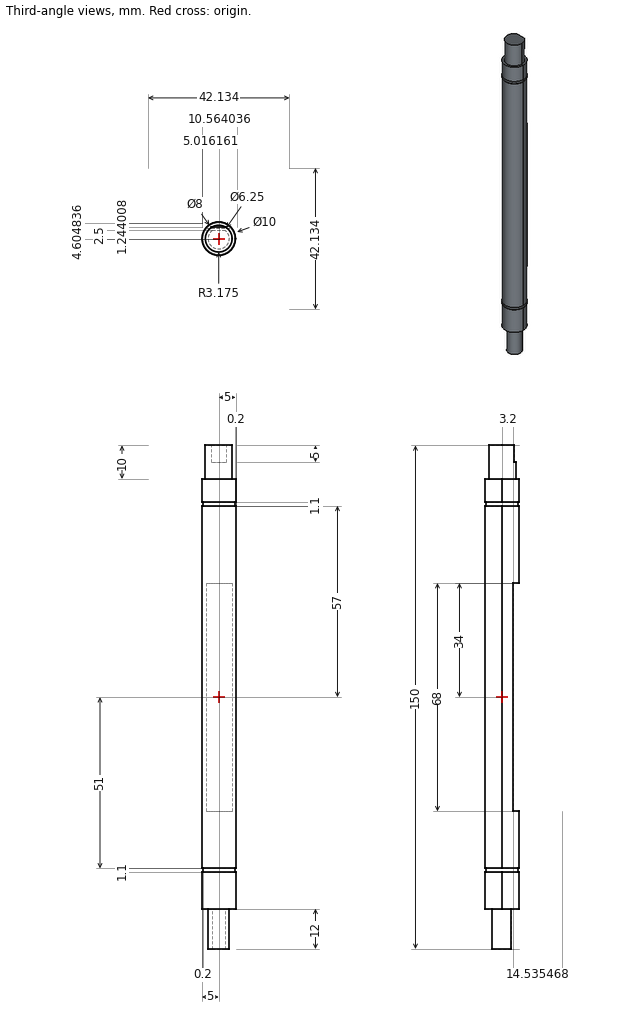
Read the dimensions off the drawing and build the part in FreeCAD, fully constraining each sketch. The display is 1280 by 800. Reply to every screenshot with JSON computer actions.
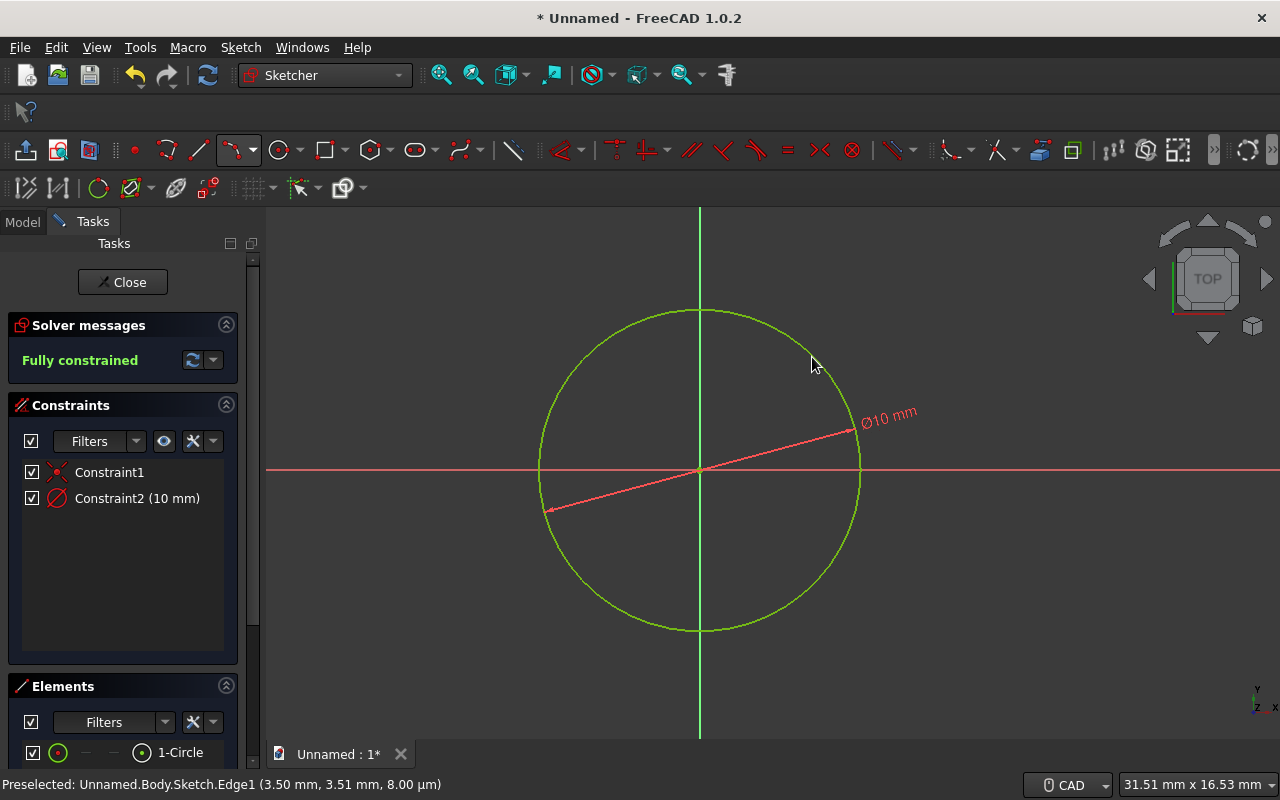
{"action": "left_click", "coordinate": [123, 282]}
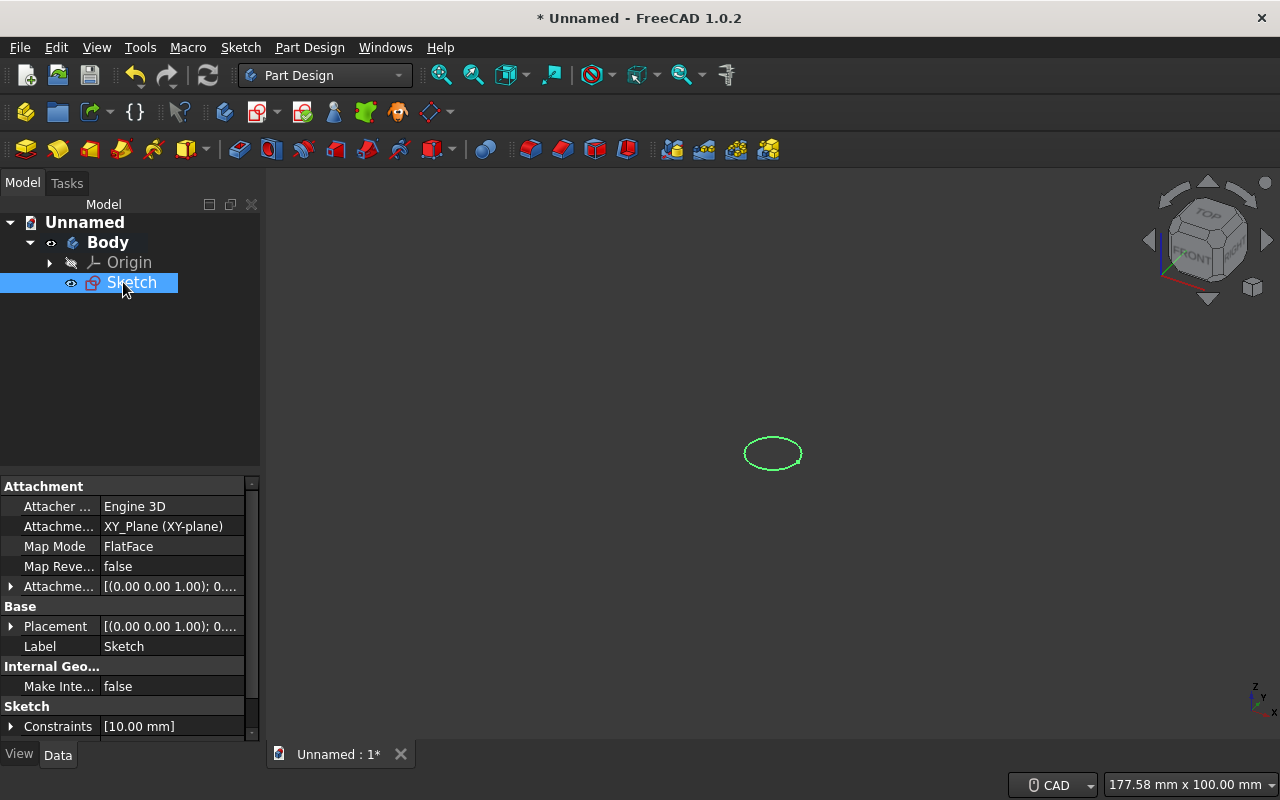
{"action": "left_click", "coordinate": [26, 150]}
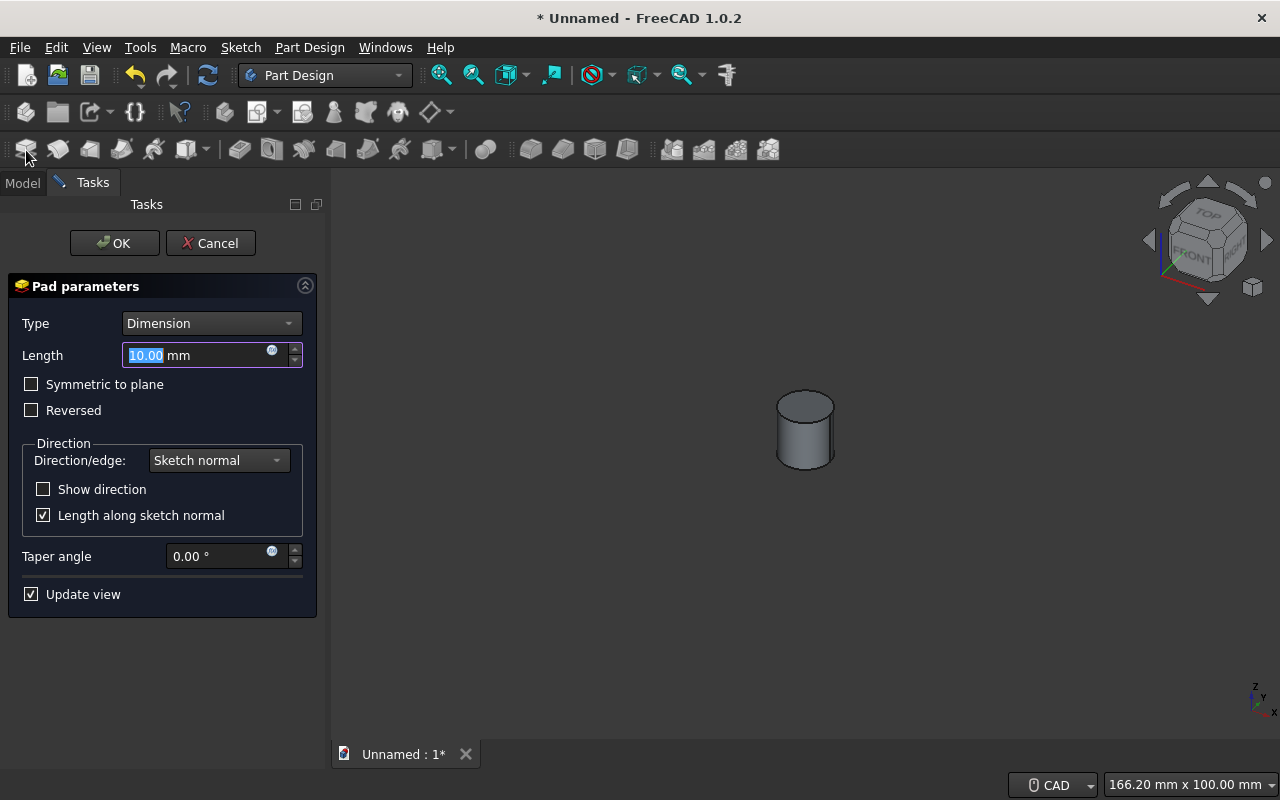
{"action": "type", "text": "150"}
{"action": "key", "text": "Tab"}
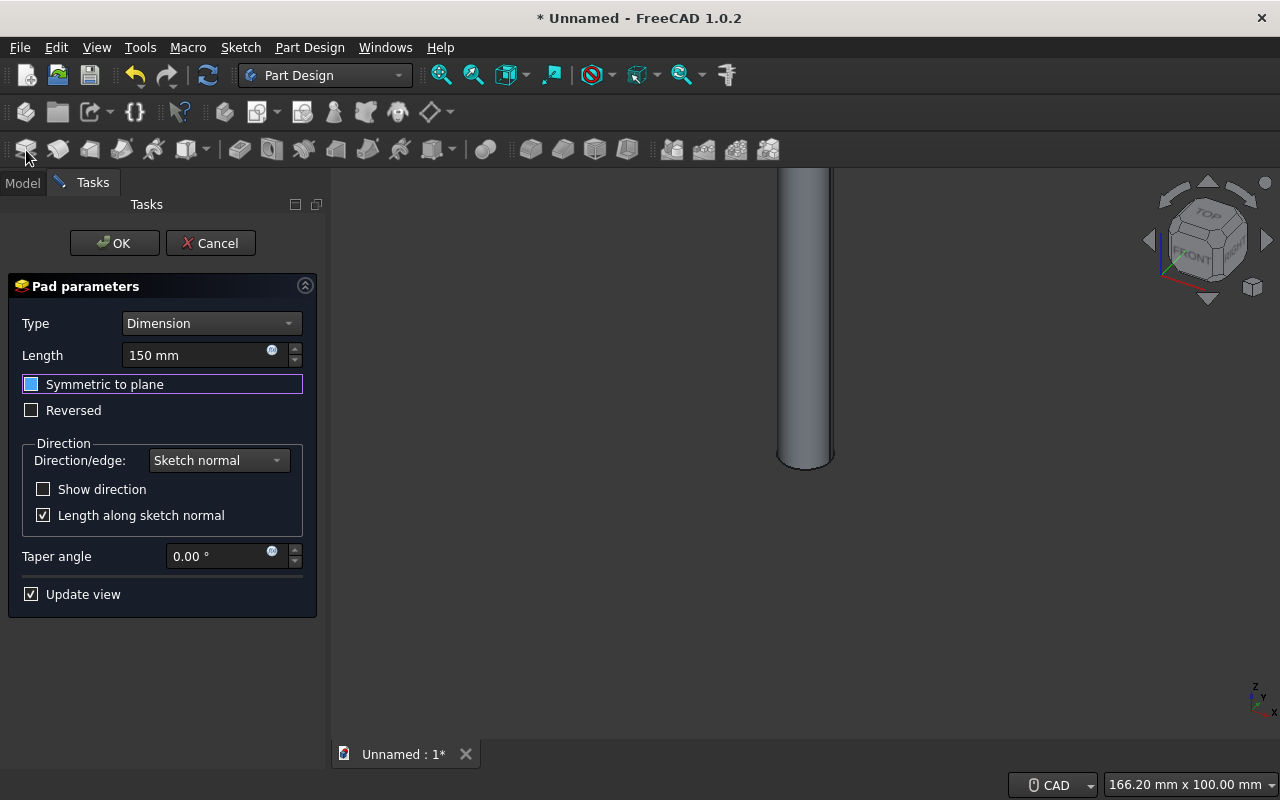
{"action": "left_click", "coordinate": [30, 384]}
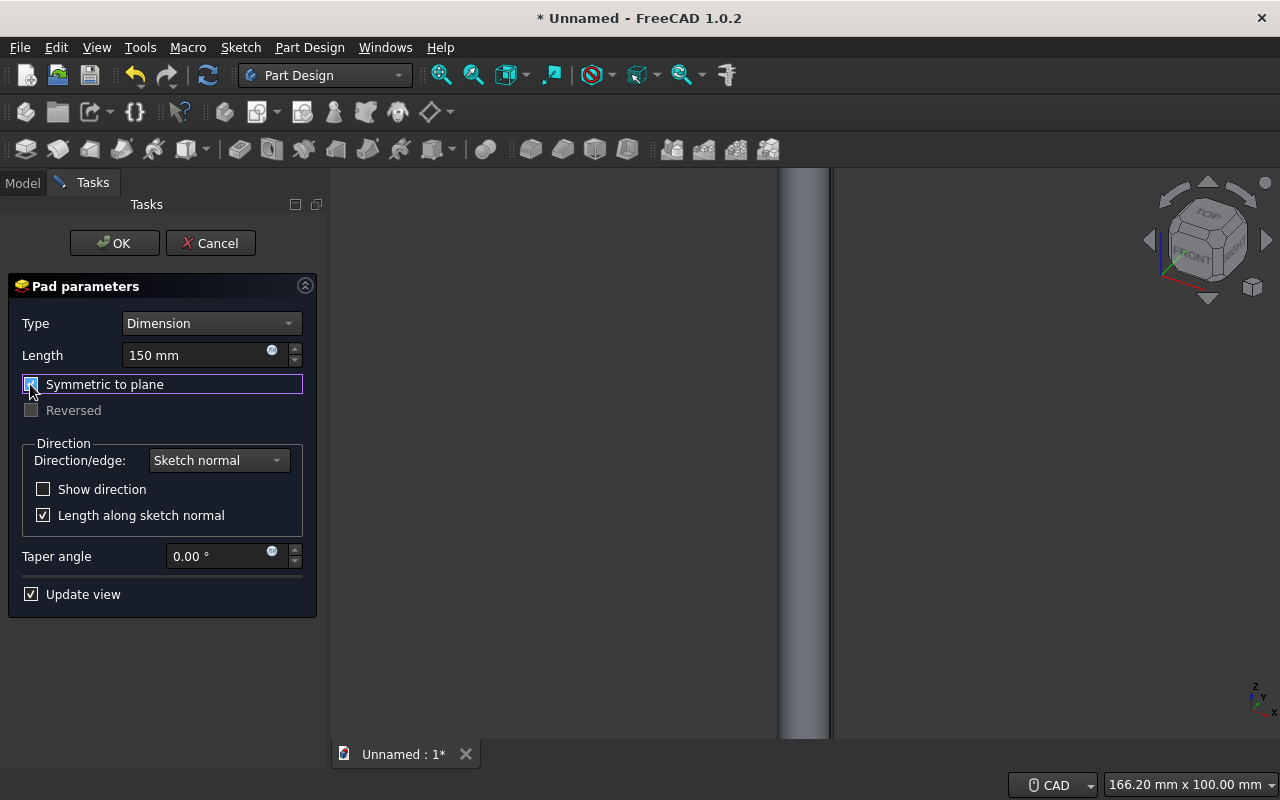
{"action": "left_click", "coordinate": [115, 243]}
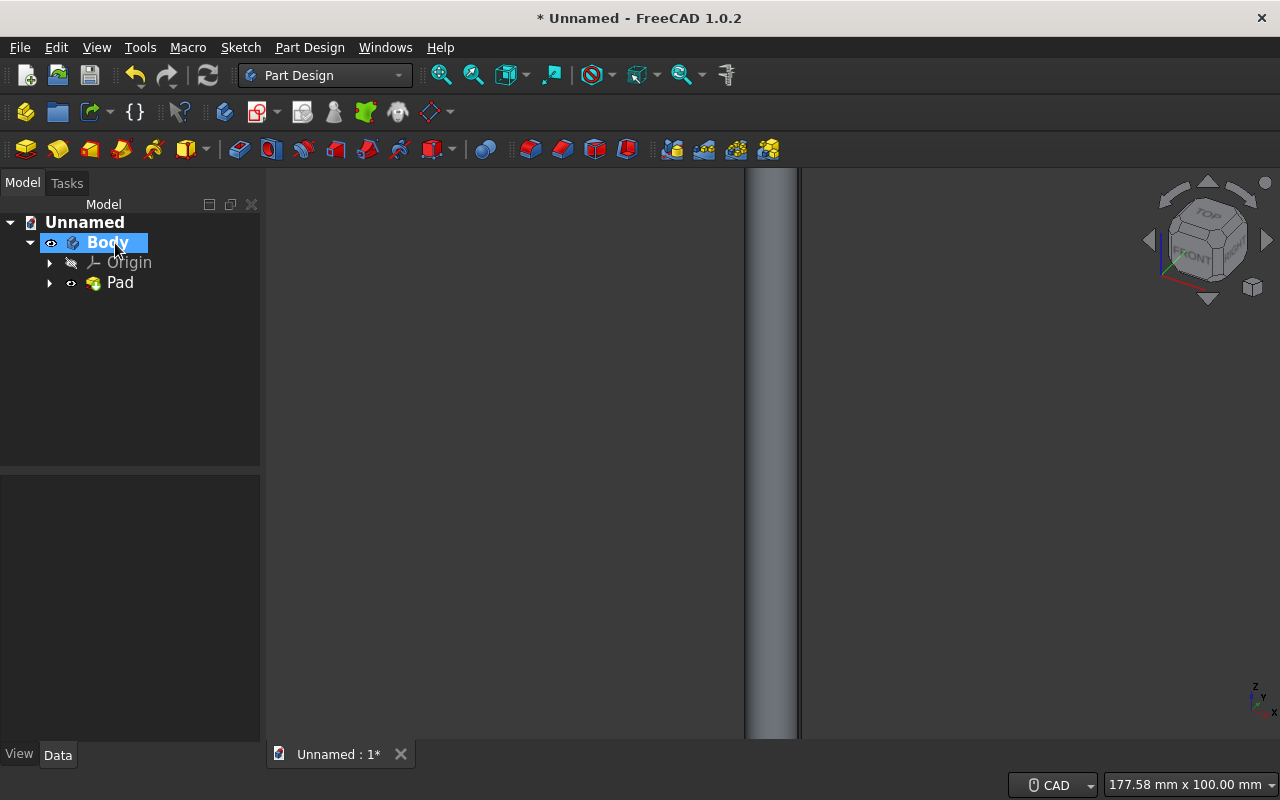
{"action": "left_click", "coordinate": [442, 76]}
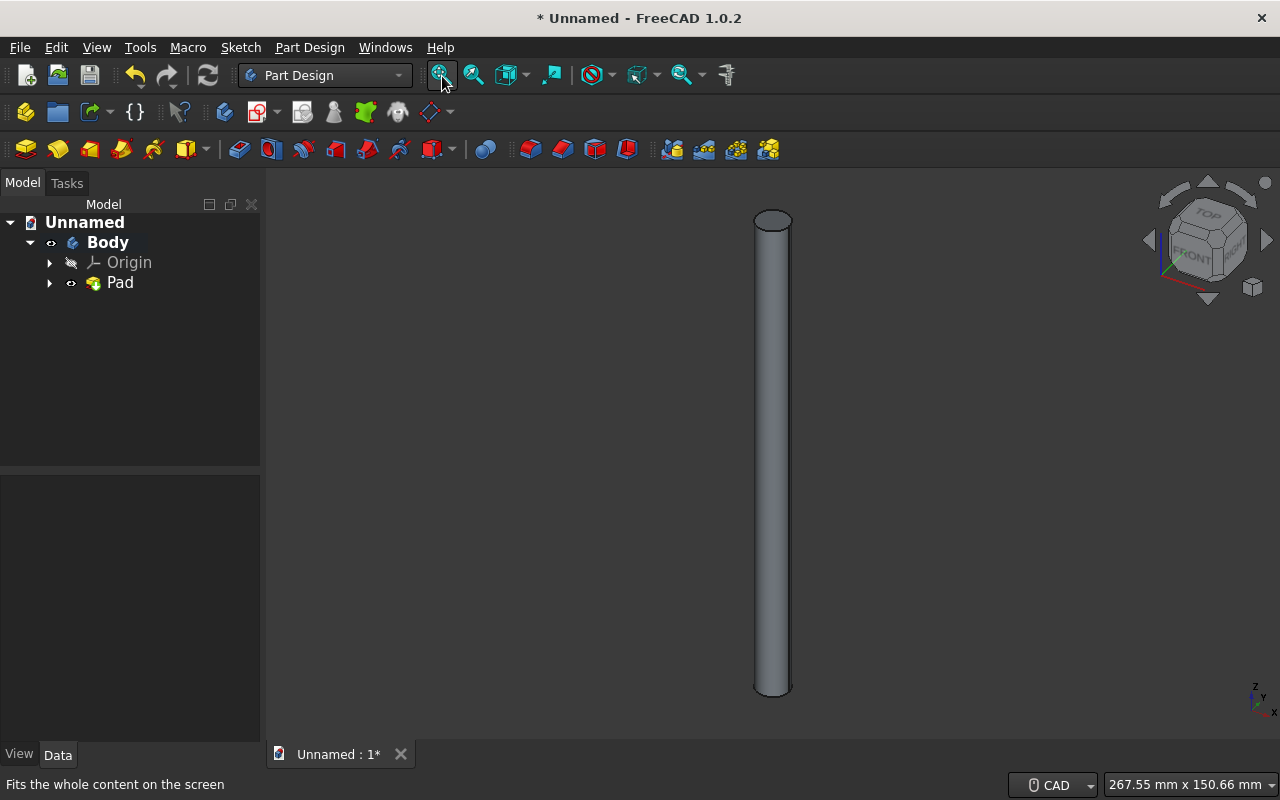
{"action": "left_click", "coordinate": [258, 112]}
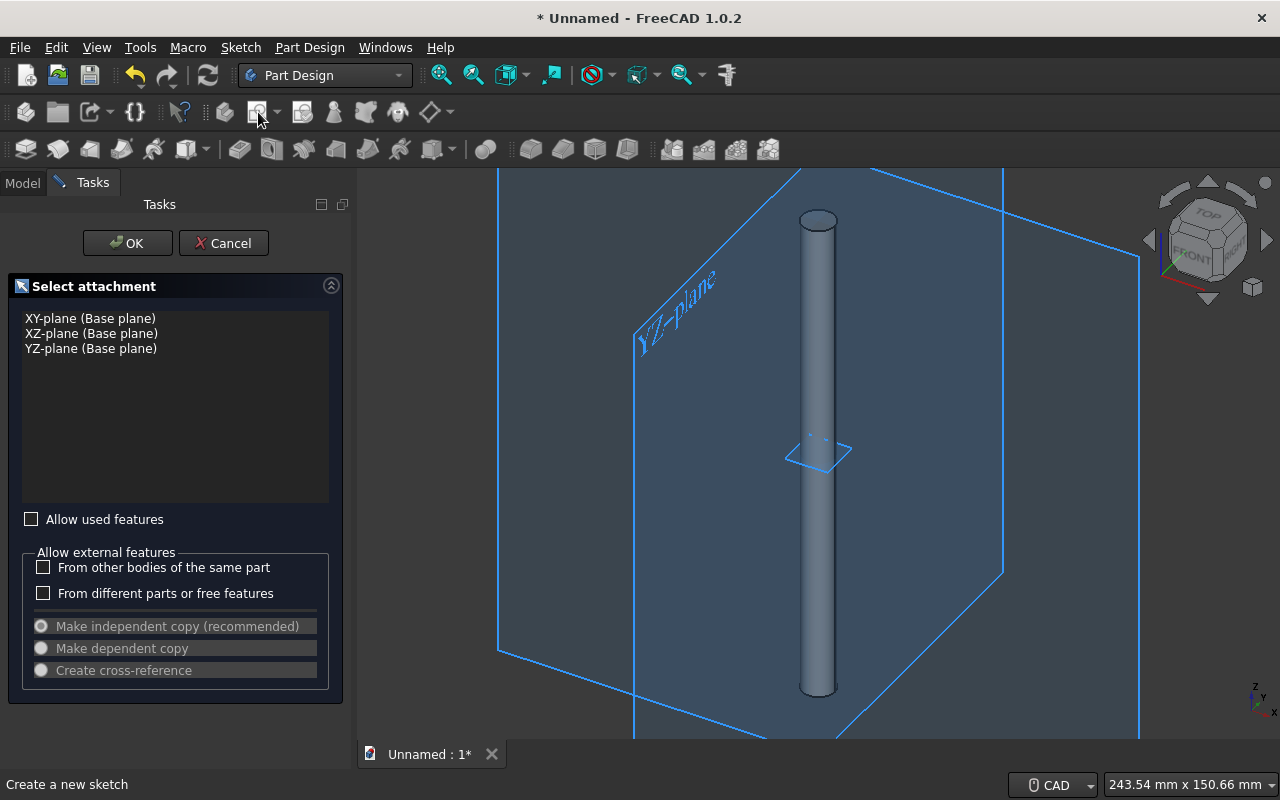
{"action": "left_click", "coordinate": [82, 348]}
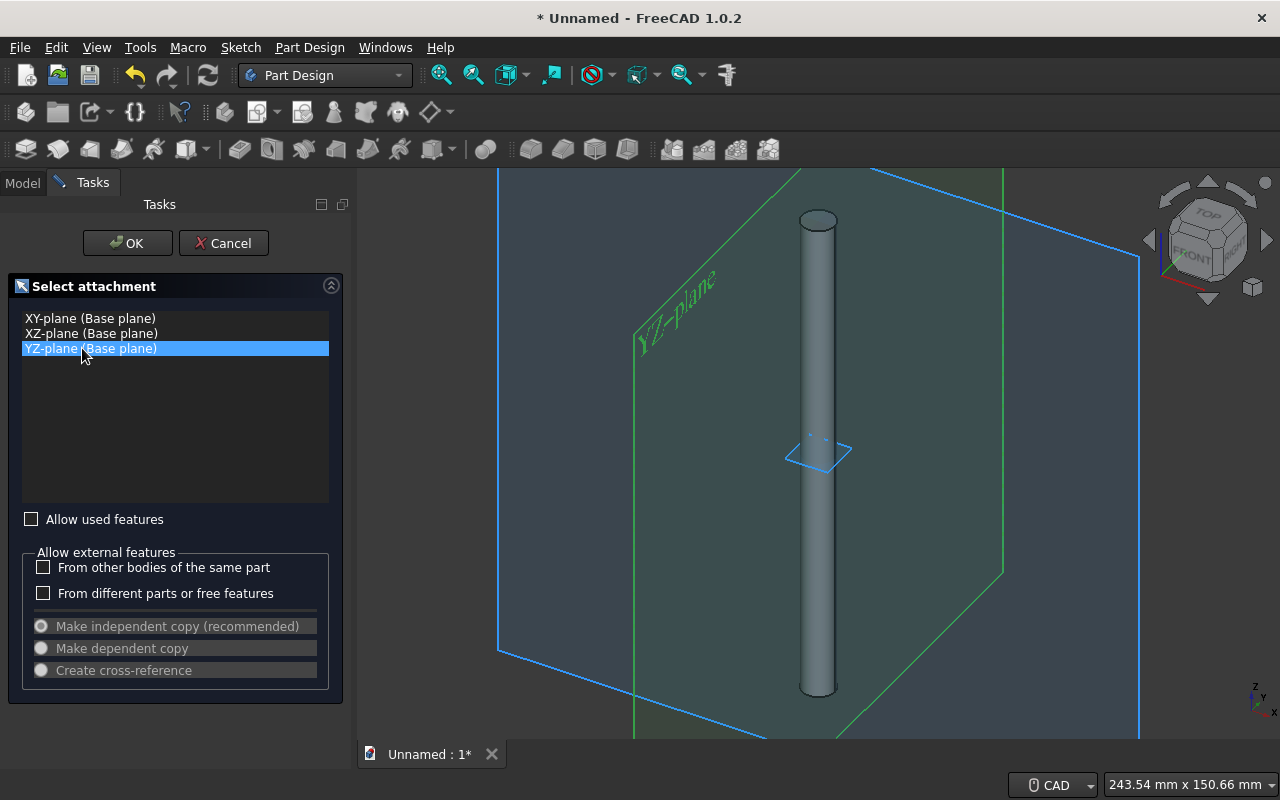
{"action": "left_click", "coordinate": [128, 243]}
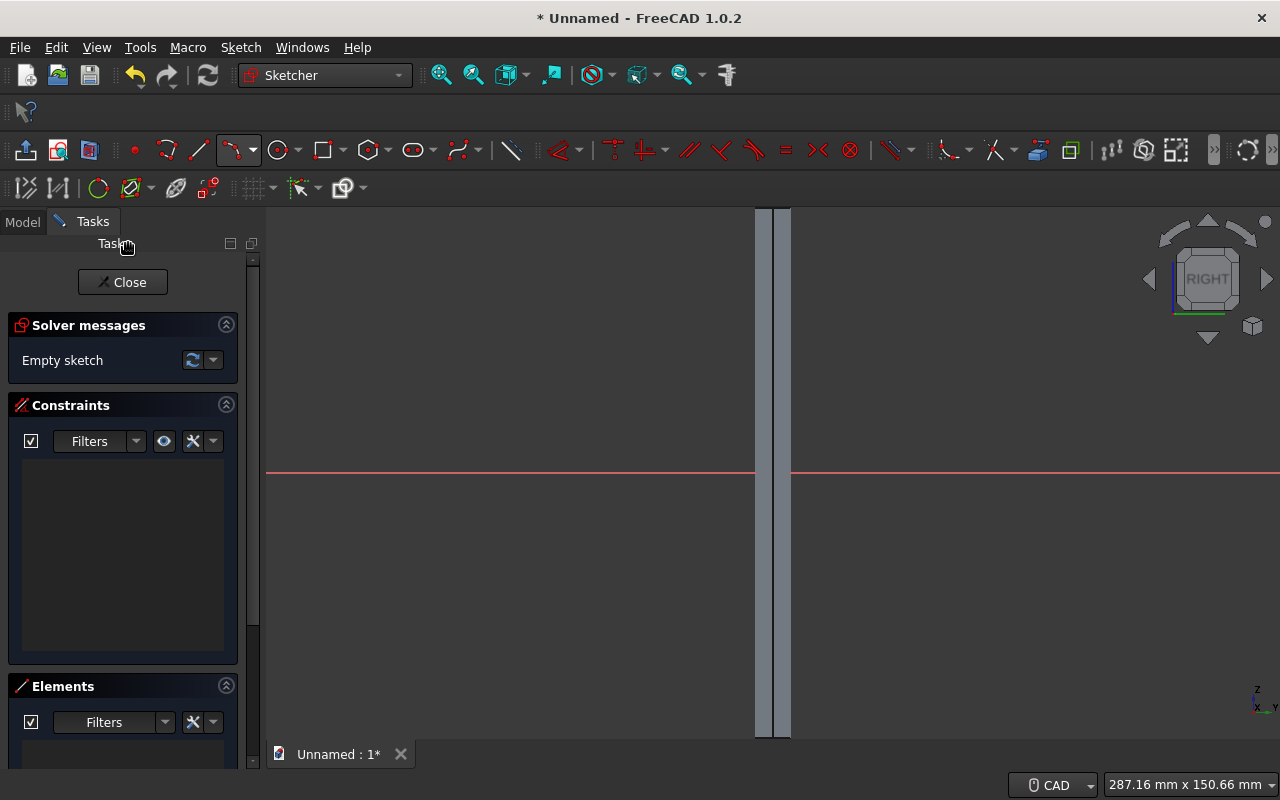
{"action": "left_click", "coordinate": [90, 150]}